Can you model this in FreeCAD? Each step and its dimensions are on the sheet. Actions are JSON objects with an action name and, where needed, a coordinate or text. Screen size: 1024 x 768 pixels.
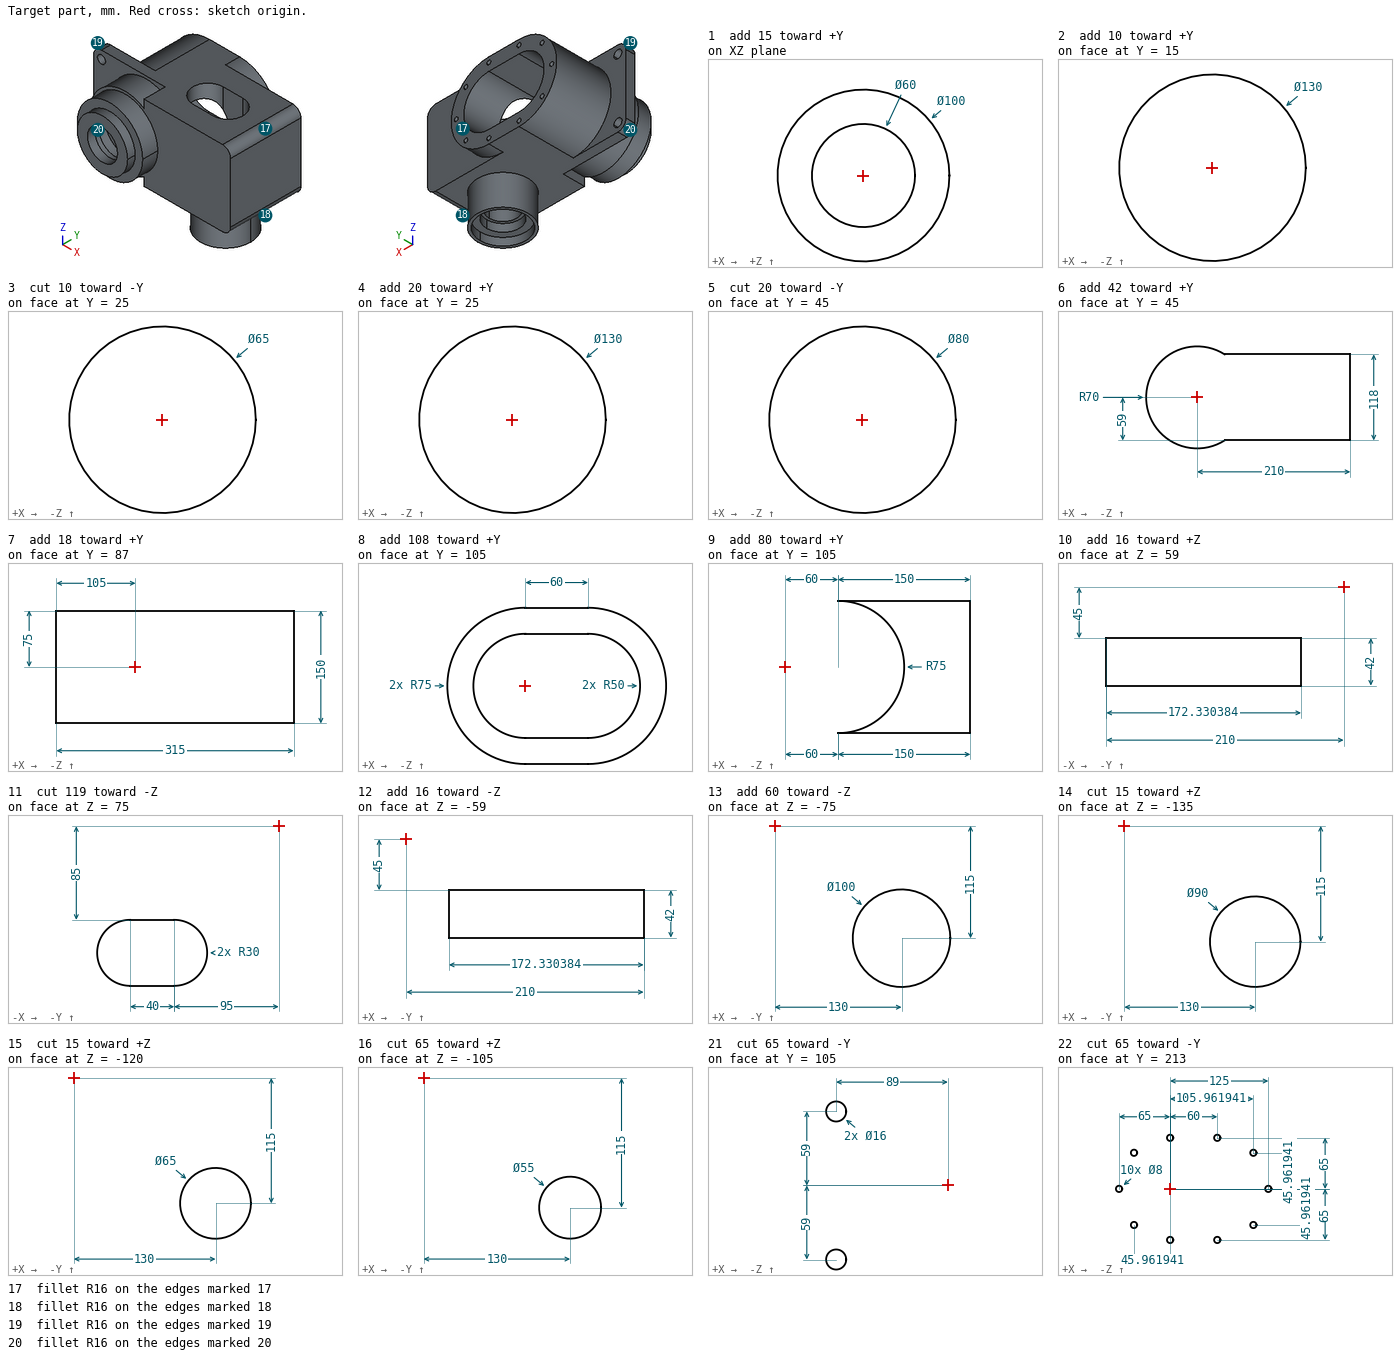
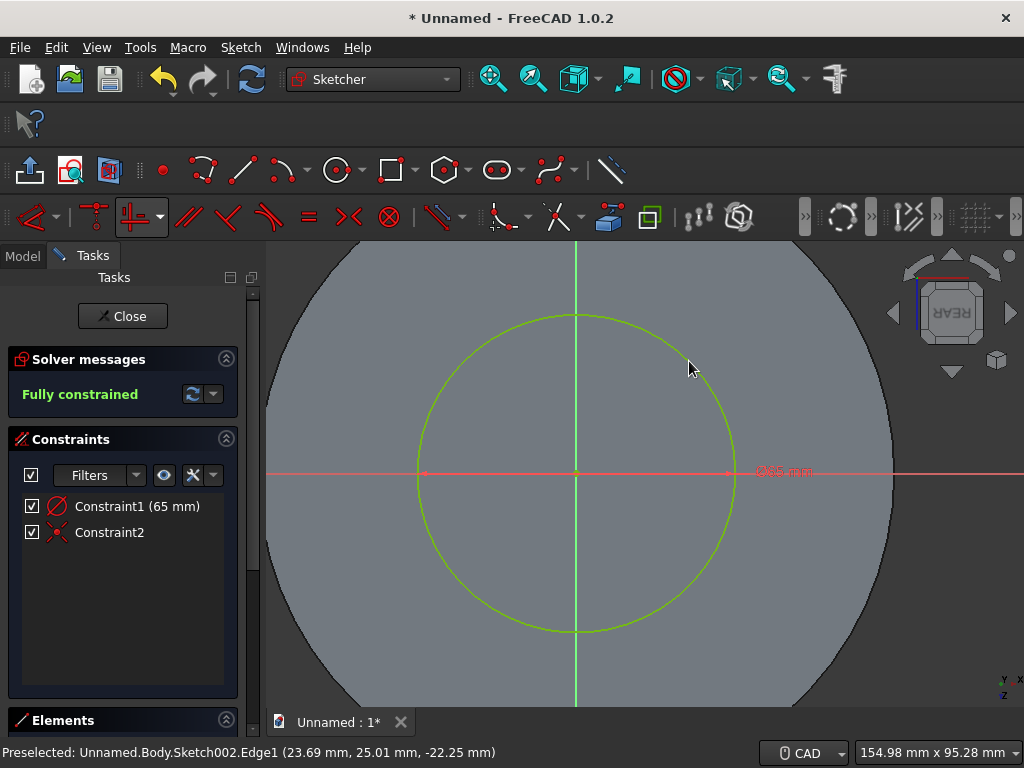
{"action": "left_click", "coordinate": [123, 316]}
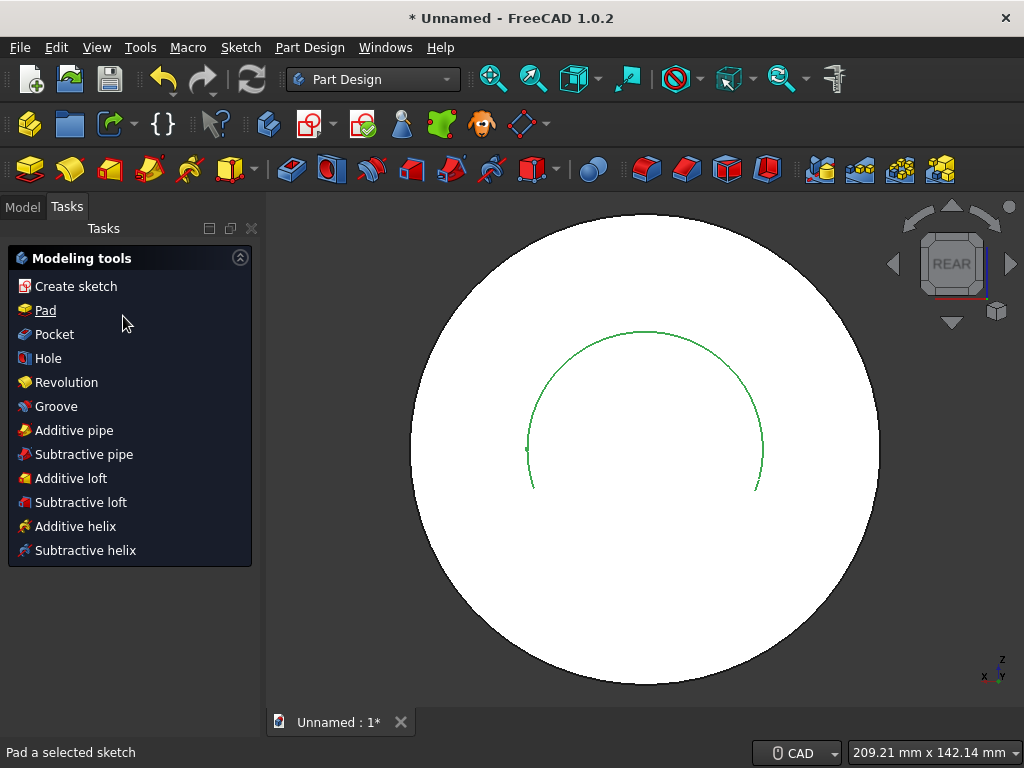
{"action": "left_click", "coordinate": [292, 170]}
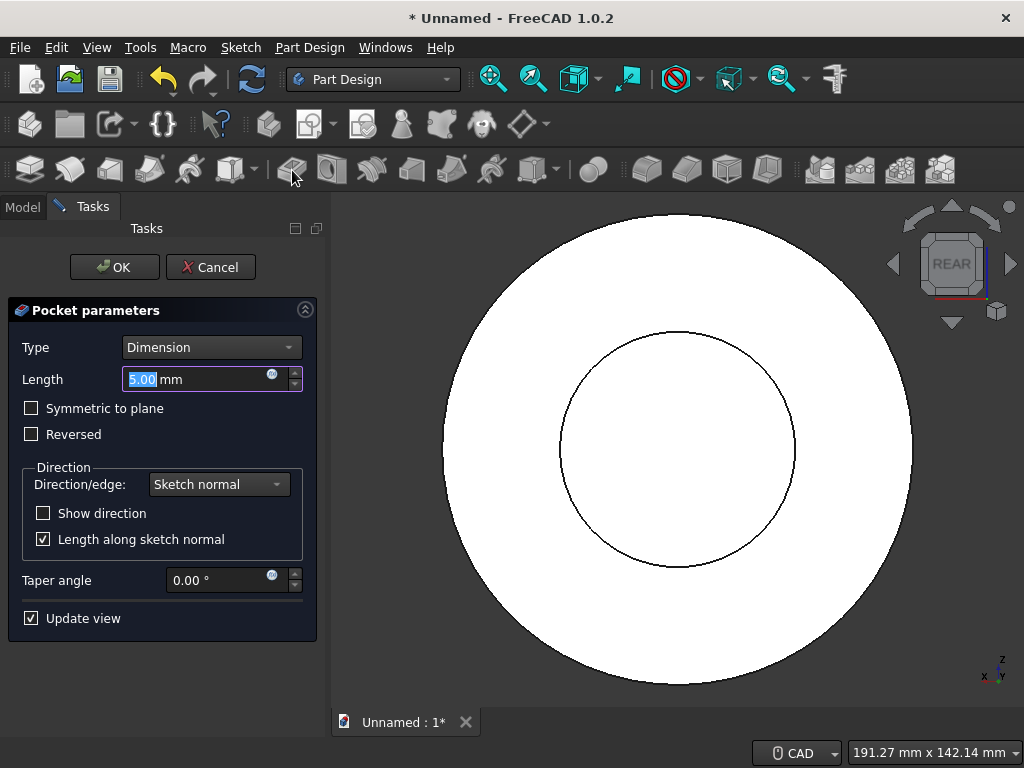
{"action": "type", "text": "10"}
{"action": "key", "text": "Tab"}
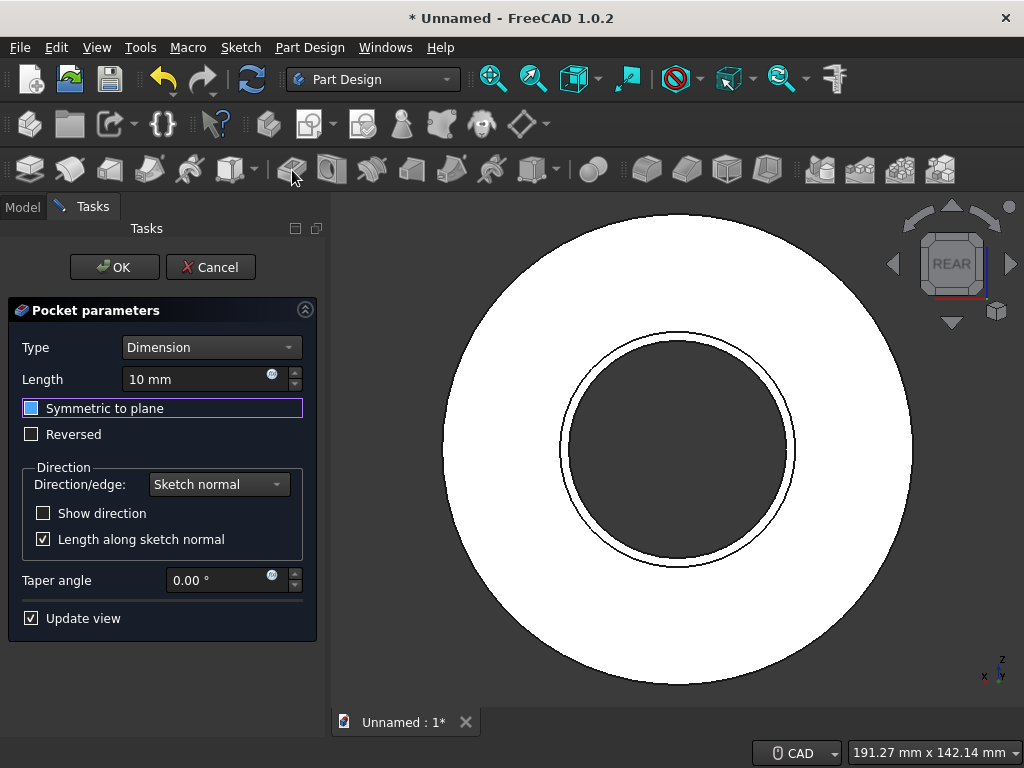
{"action": "left_click", "coordinate": [115, 267]}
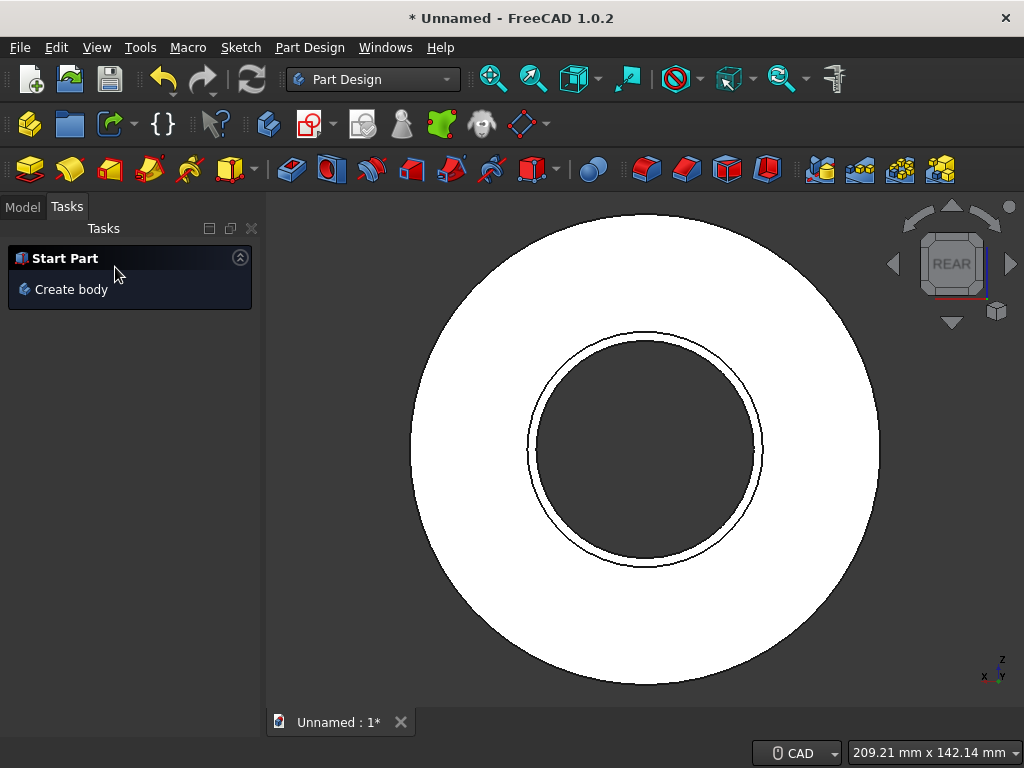
{"action": "left_click", "coordinate": [511, 314]}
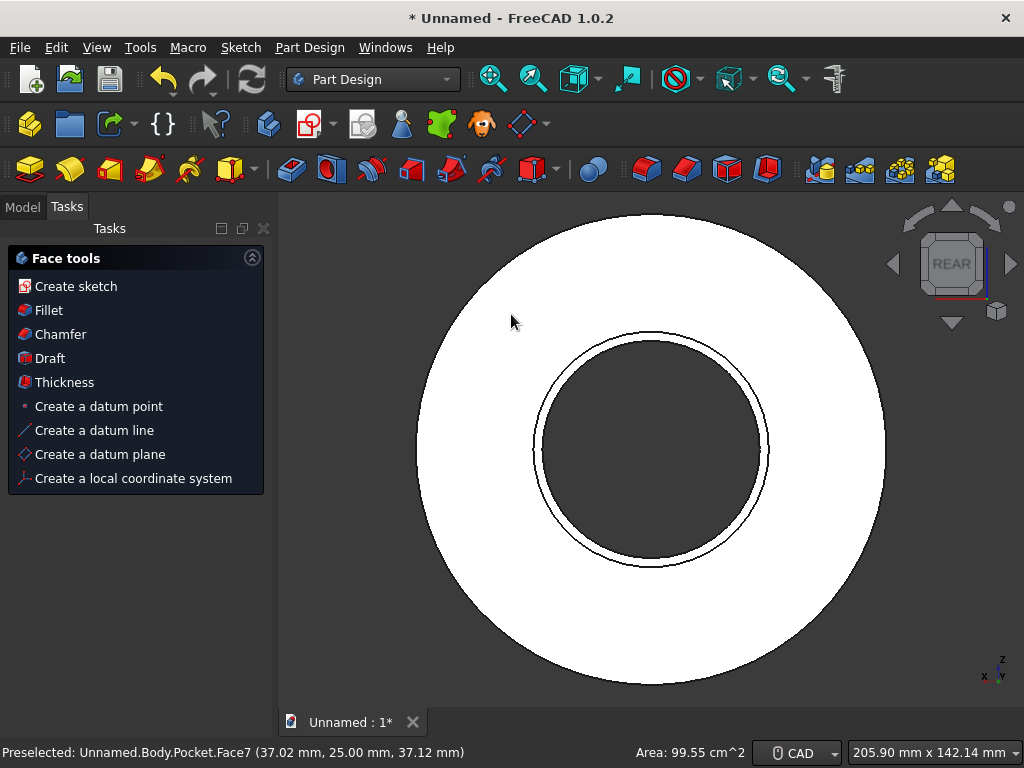
{"action": "left_click", "coordinate": [310, 124]}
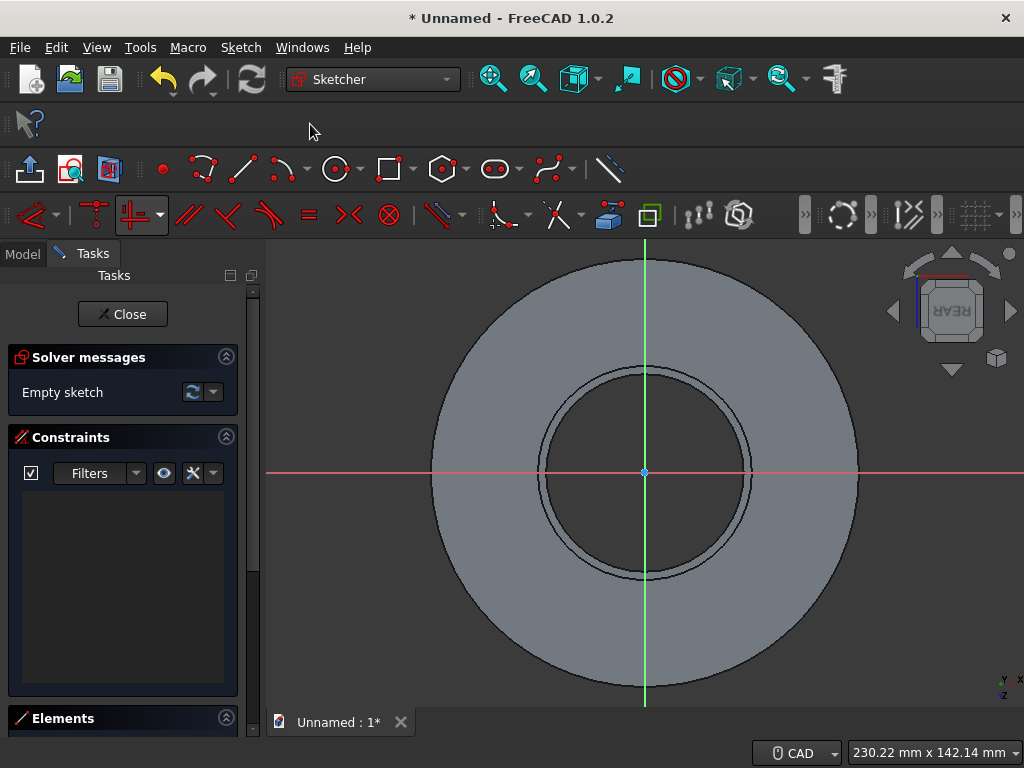
{"action": "scroll", "coordinate": [437, 473], "scroll_direction": "down", "scroll_amount": 2}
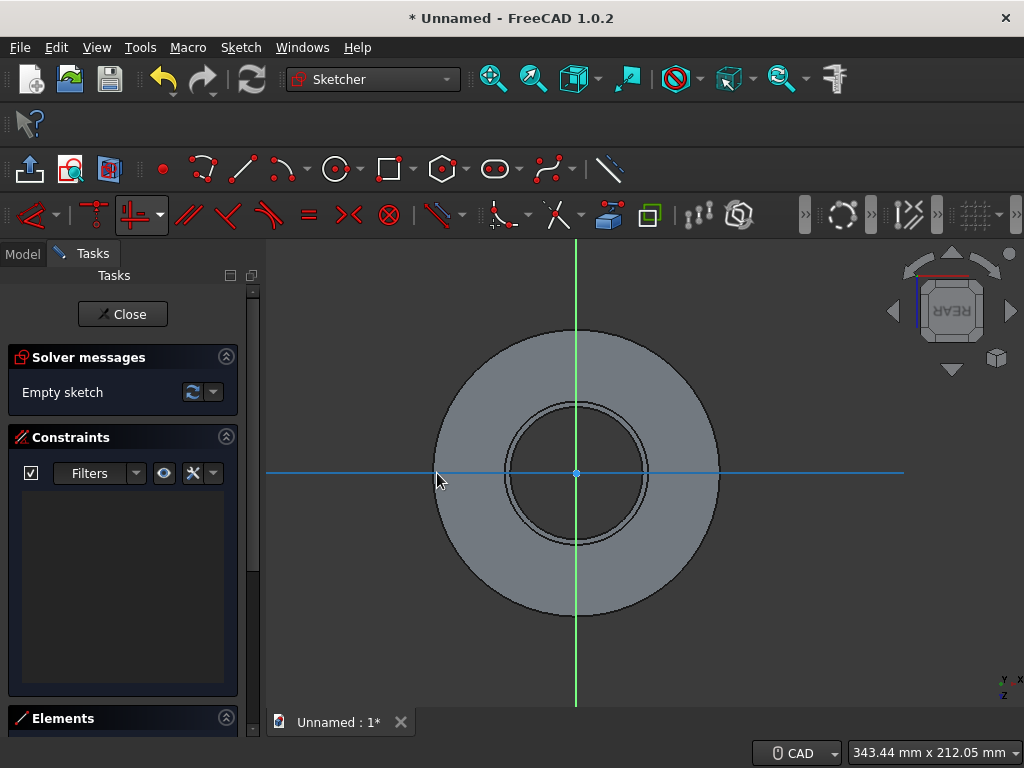
{"action": "left_click", "coordinate": [336, 170]}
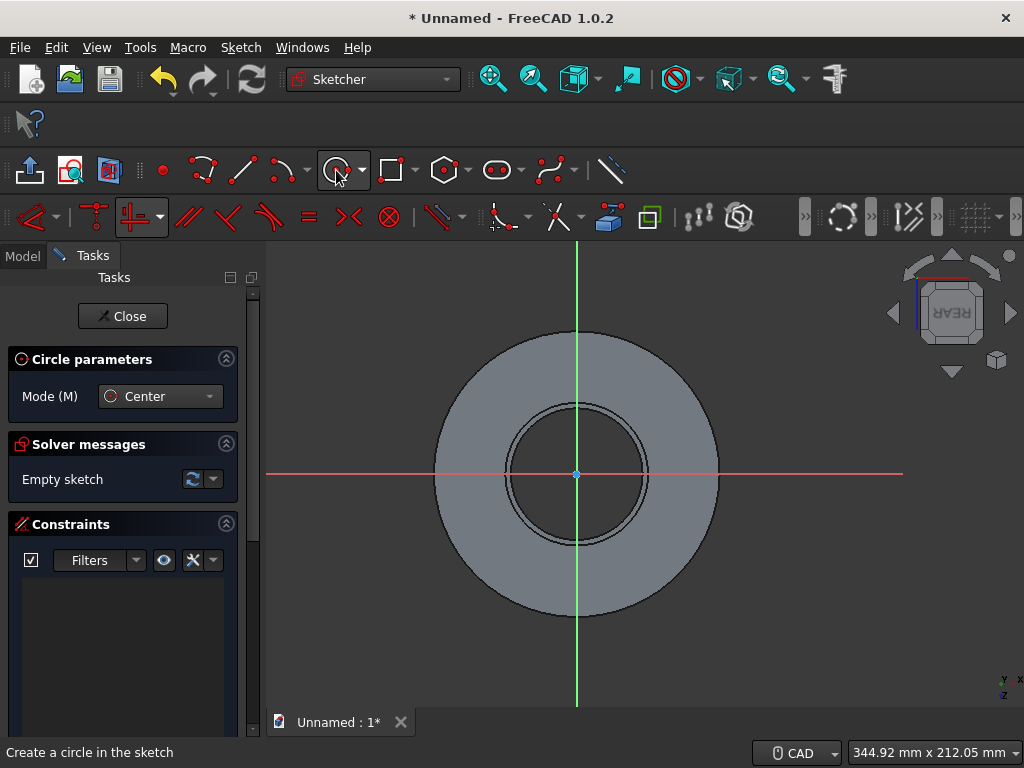
{"action": "left_click", "coordinate": [577, 474]}
{"action": "mouse_move", "coordinate": [678, 373]}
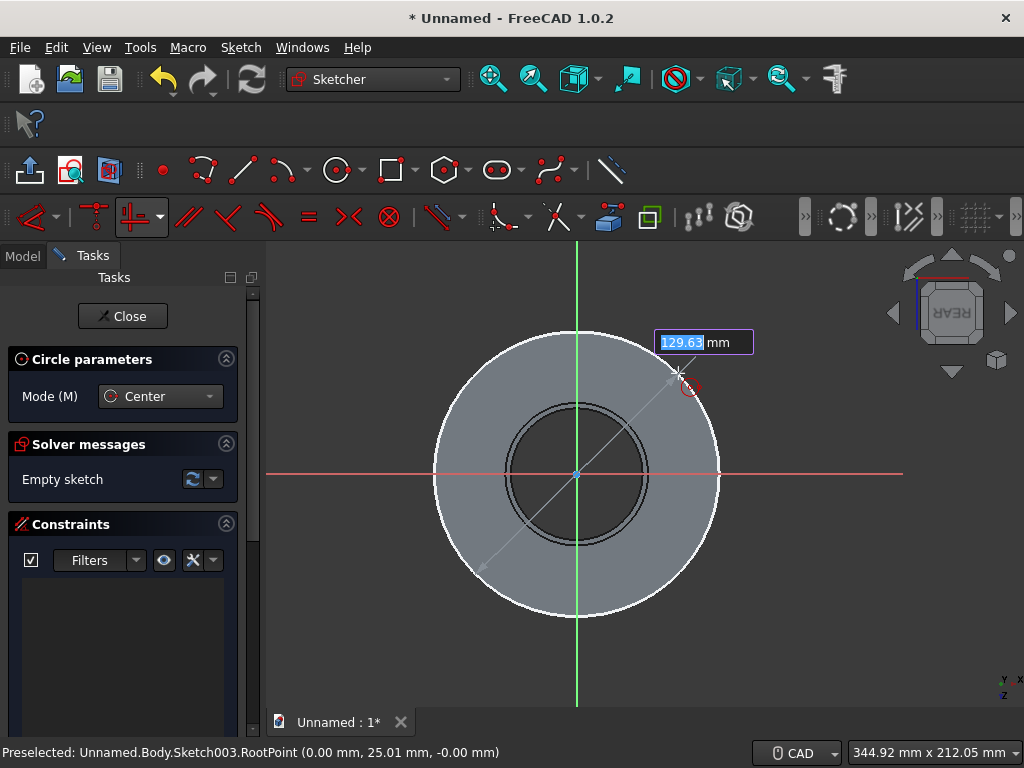
{"action": "type", "text": "130"}
{"action": "key", "text": "Return"}
{"action": "key", "text": "Escape"}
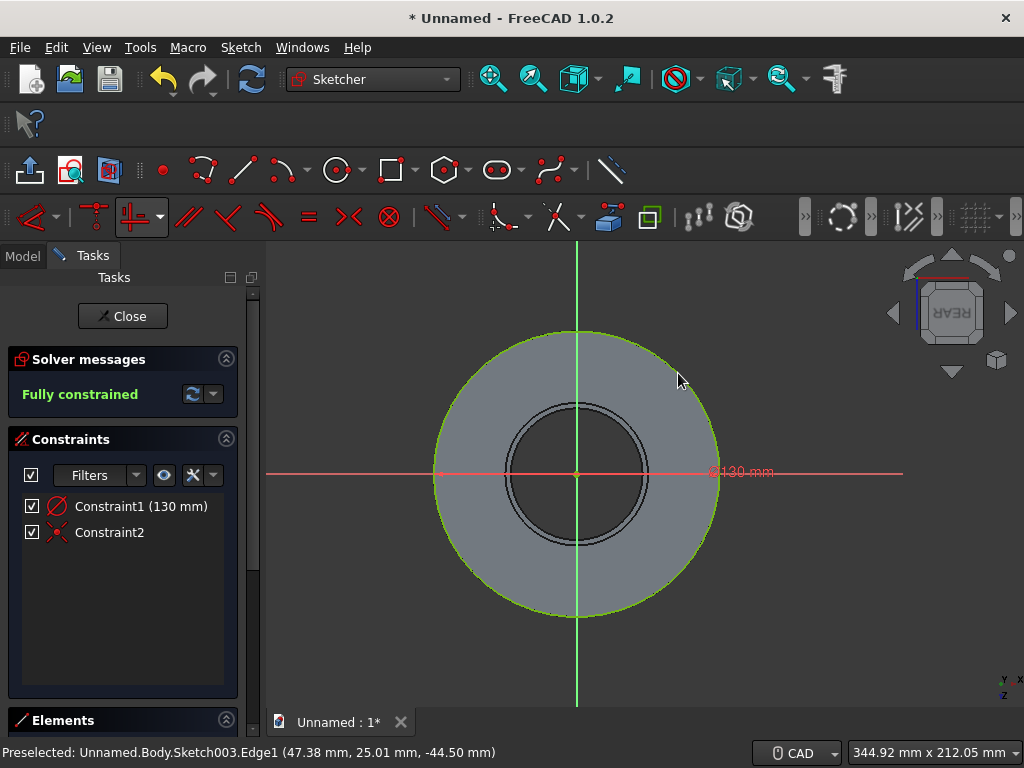
{"action": "left_click", "coordinate": [123, 316]}